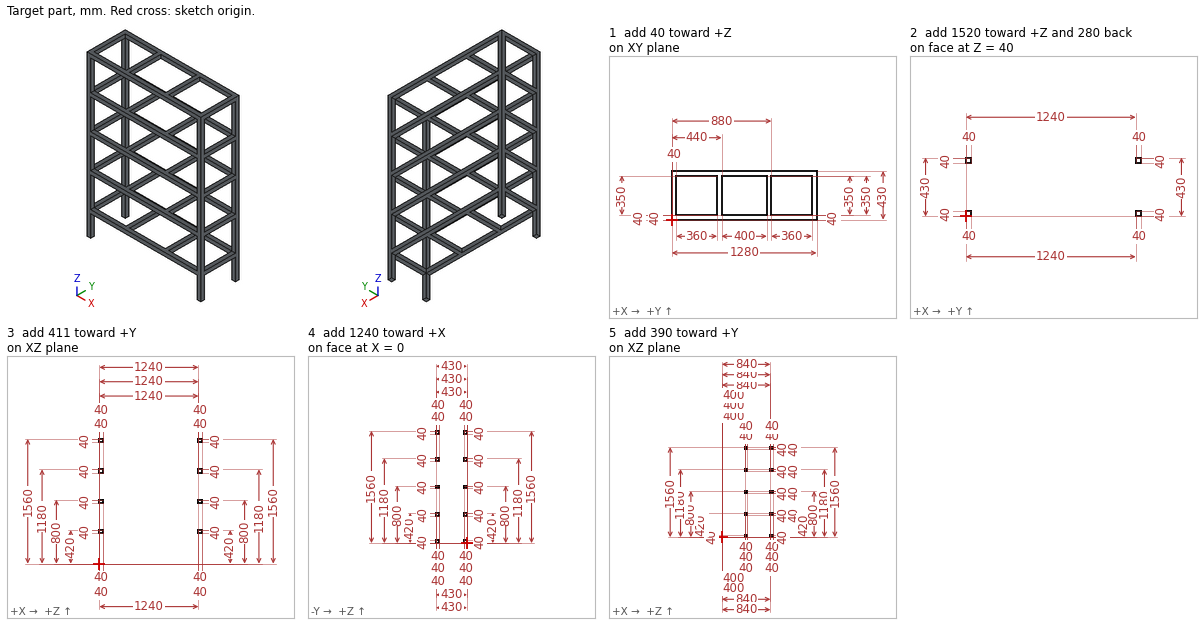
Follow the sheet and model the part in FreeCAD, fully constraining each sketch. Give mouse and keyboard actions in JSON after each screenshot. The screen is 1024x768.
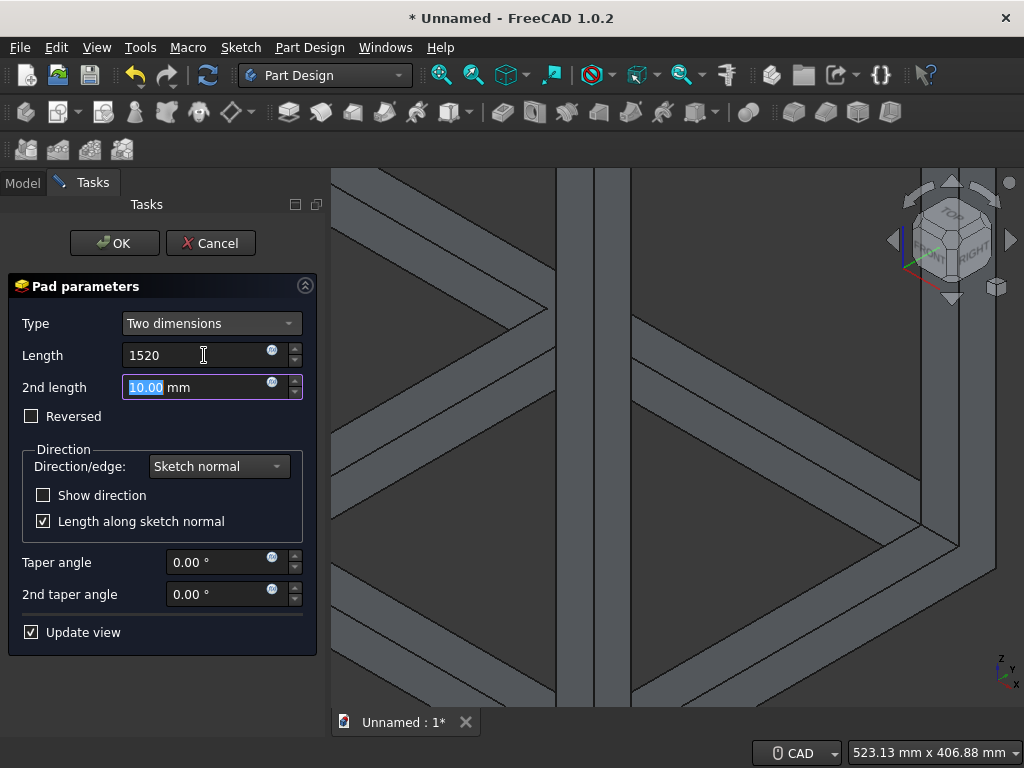
{"action": "type", "text": "280"}
{"action": "key", "text": "Tab"}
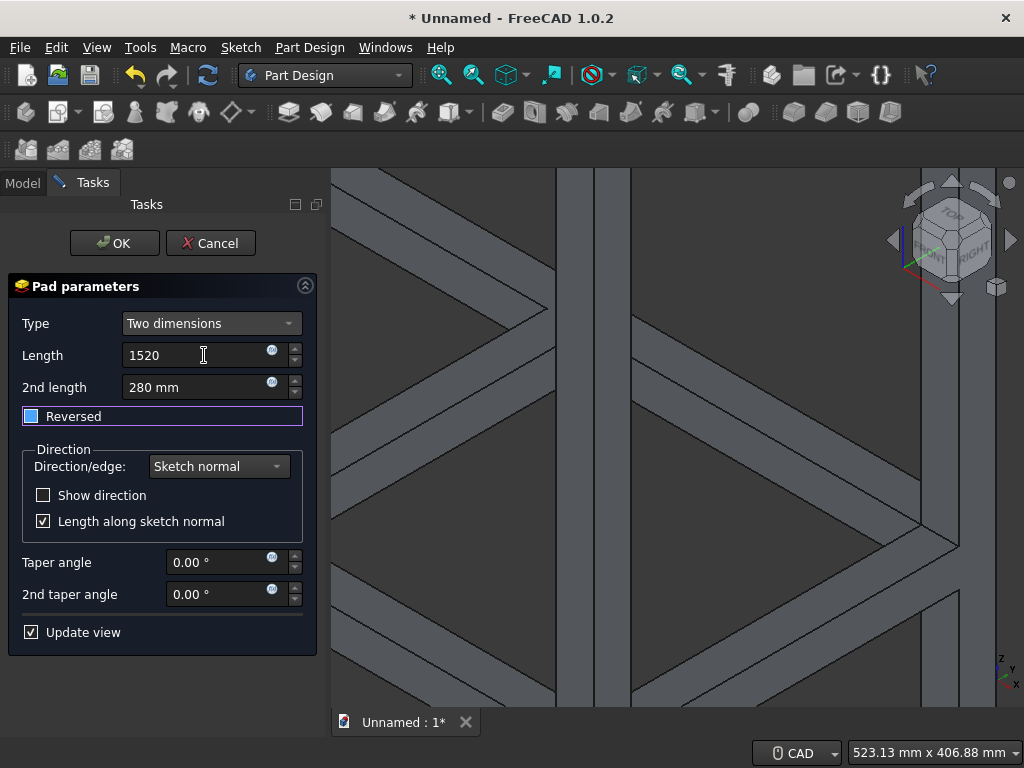
{"action": "left_click", "coordinate": [115, 243]}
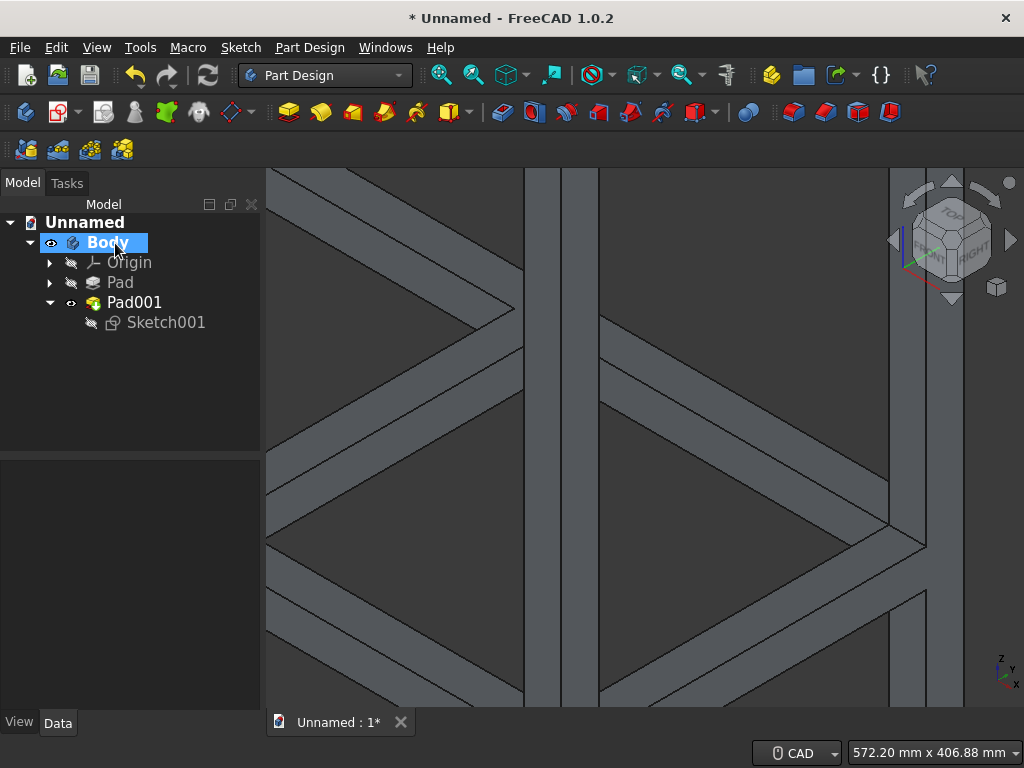
{"action": "left_click", "coordinate": [442, 76]}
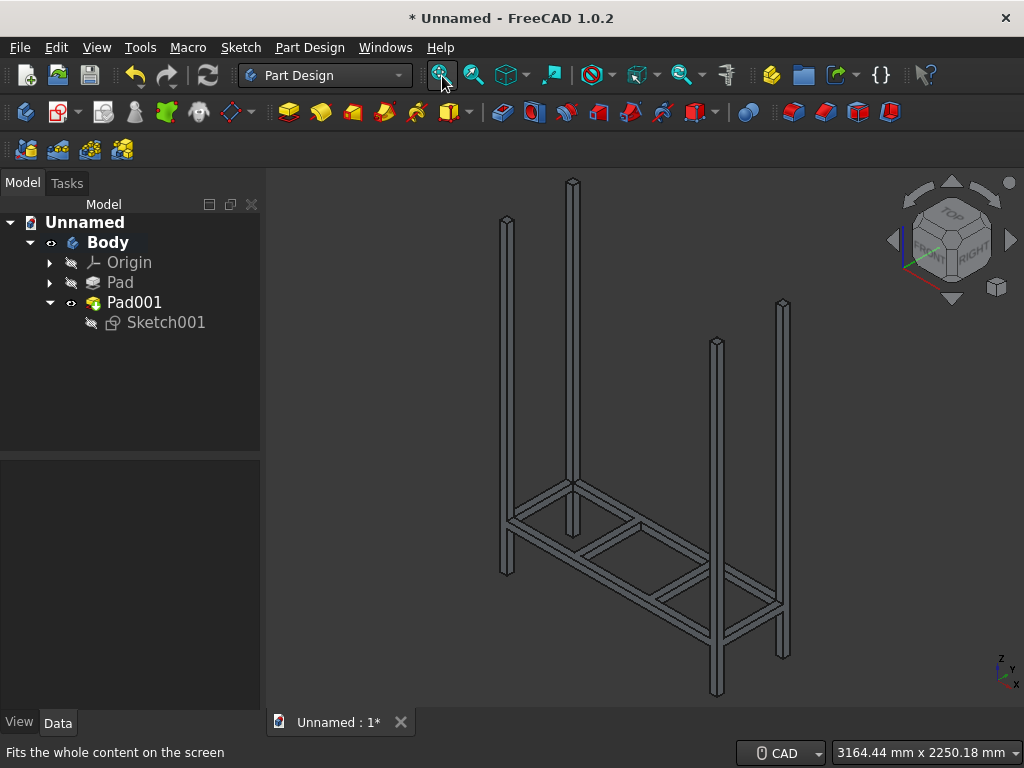
{"action": "left_click", "coordinate": [58, 112]}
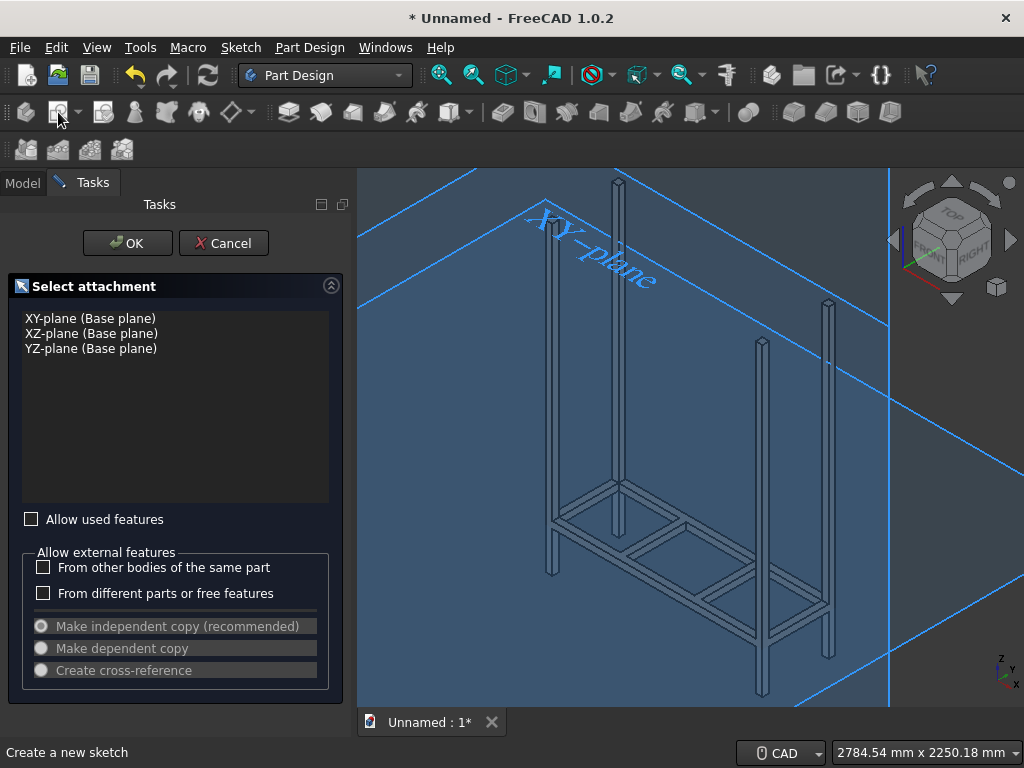
{"action": "left_click", "coordinate": [82, 334]}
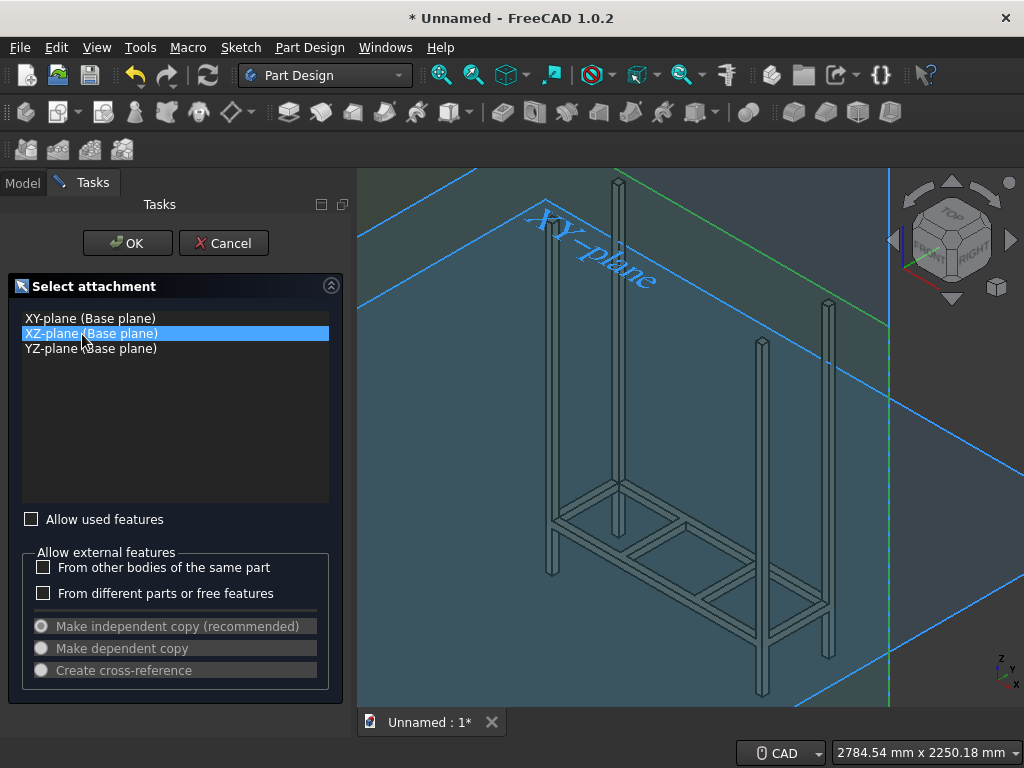
{"action": "left_click", "coordinate": [128, 243]}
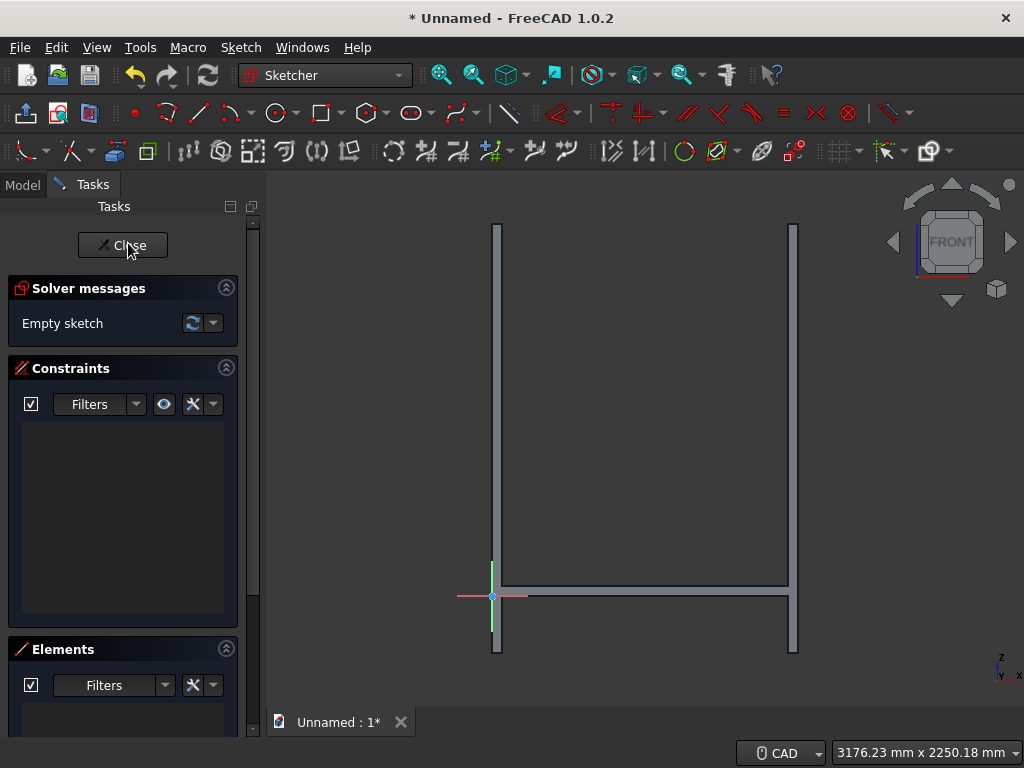
{"action": "left_click", "coordinate": [322, 114]}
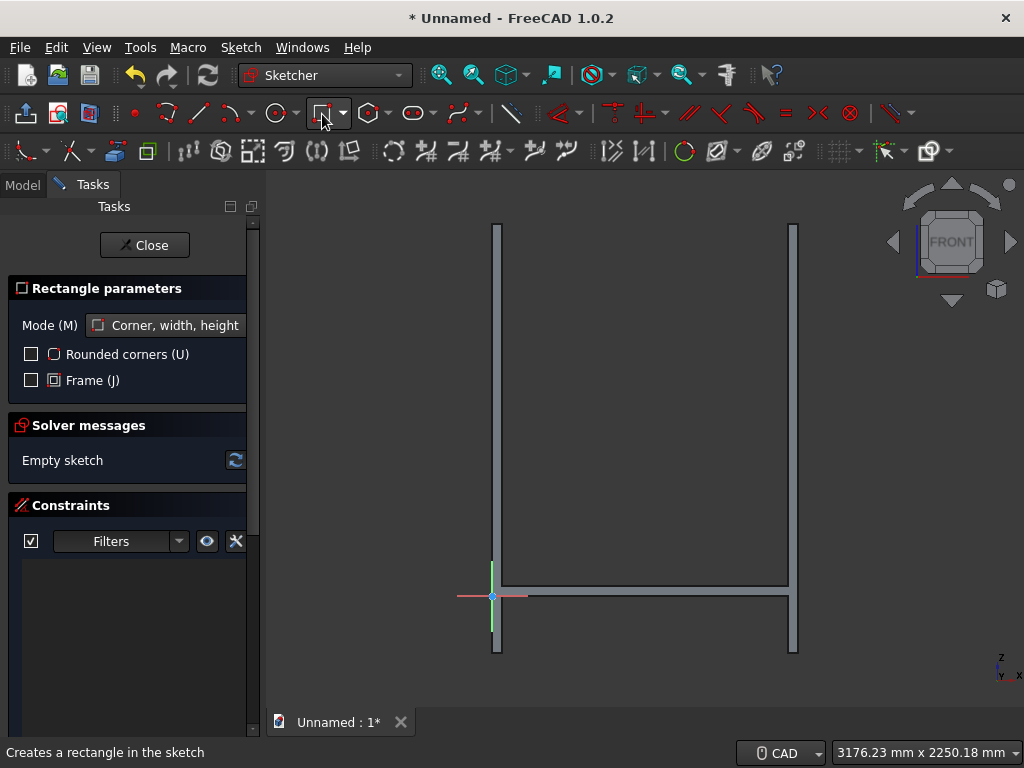
{"action": "scroll", "coordinate": [492, 496], "scroll_direction": "up", "scroll_amount": 3}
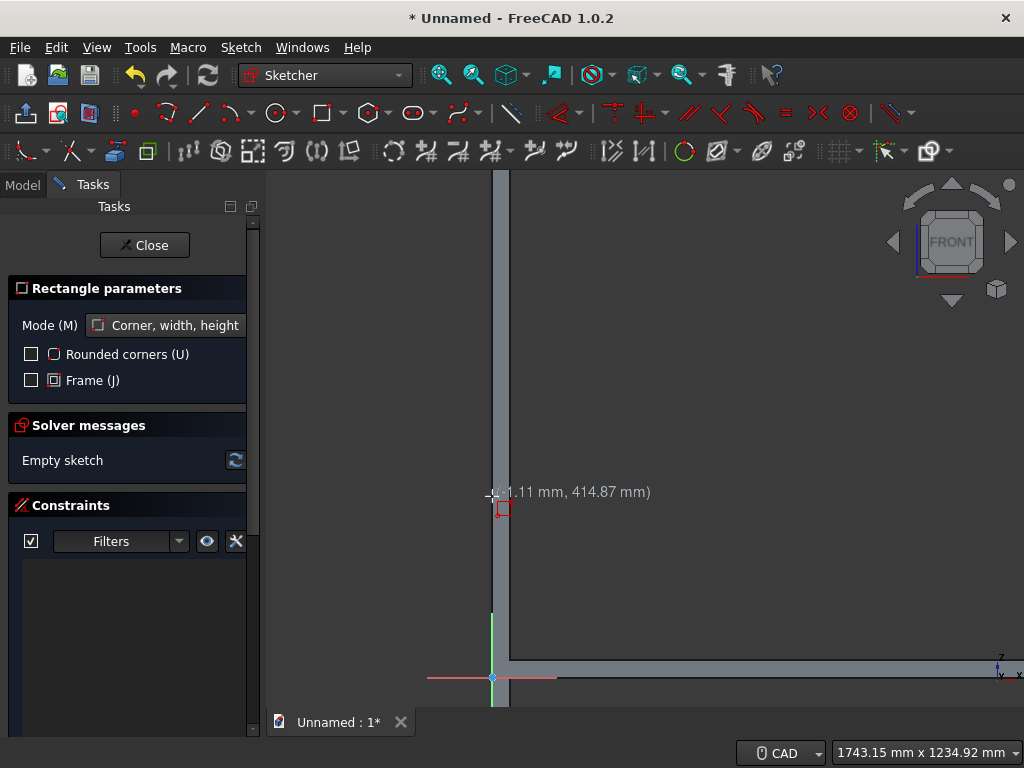
{"action": "left_click", "coordinate": [492, 495]}
{"action": "mouse_move", "coordinate": [510, 512]}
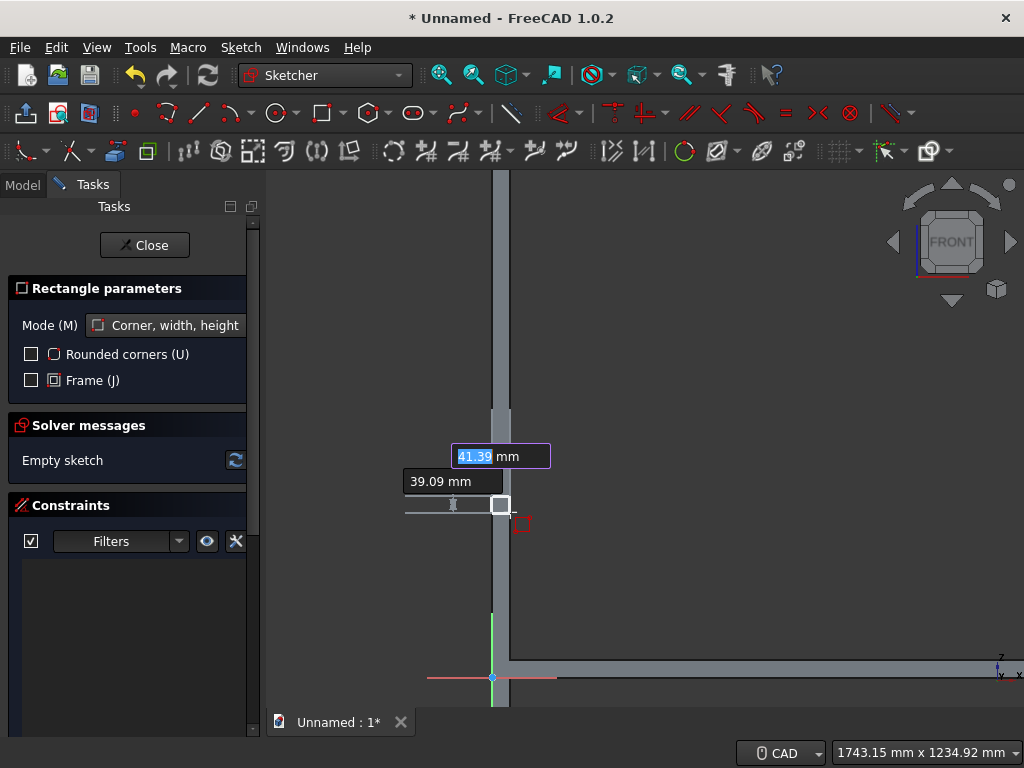
{"action": "type", "text": "40"}
{"action": "key", "text": "Tab"}
{"action": "type", "text": "40"}
{"action": "key", "text": "Return"}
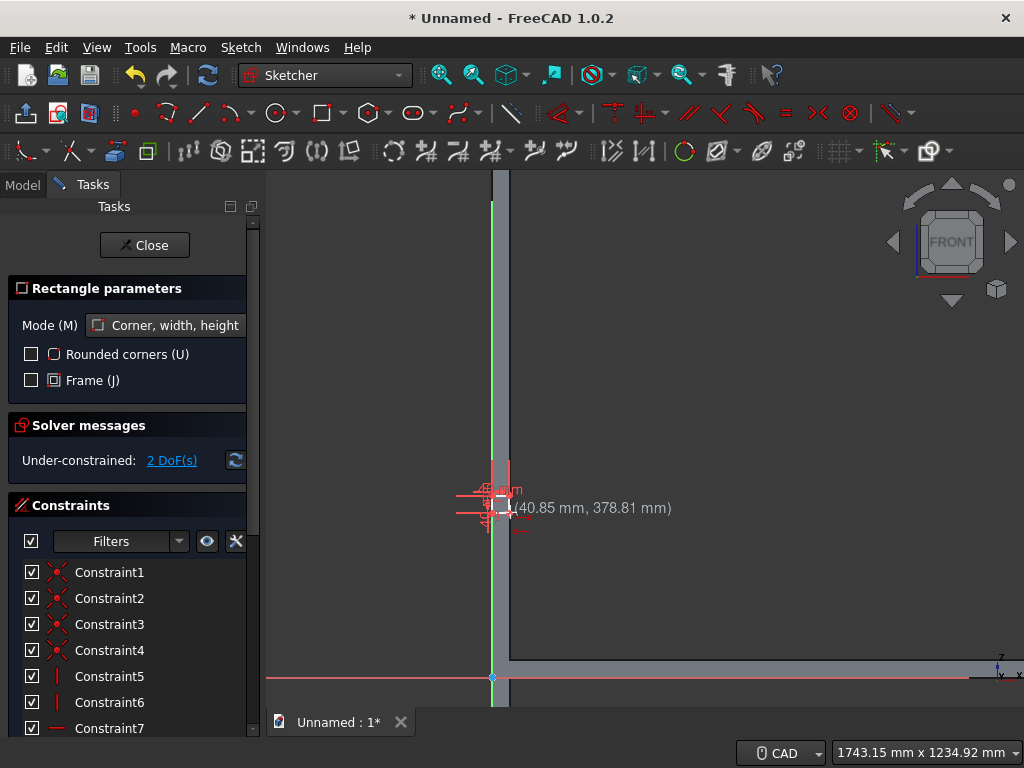
{"action": "scroll", "coordinate": [340, 560], "scroll_direction": "down", "scroll_amount": 3}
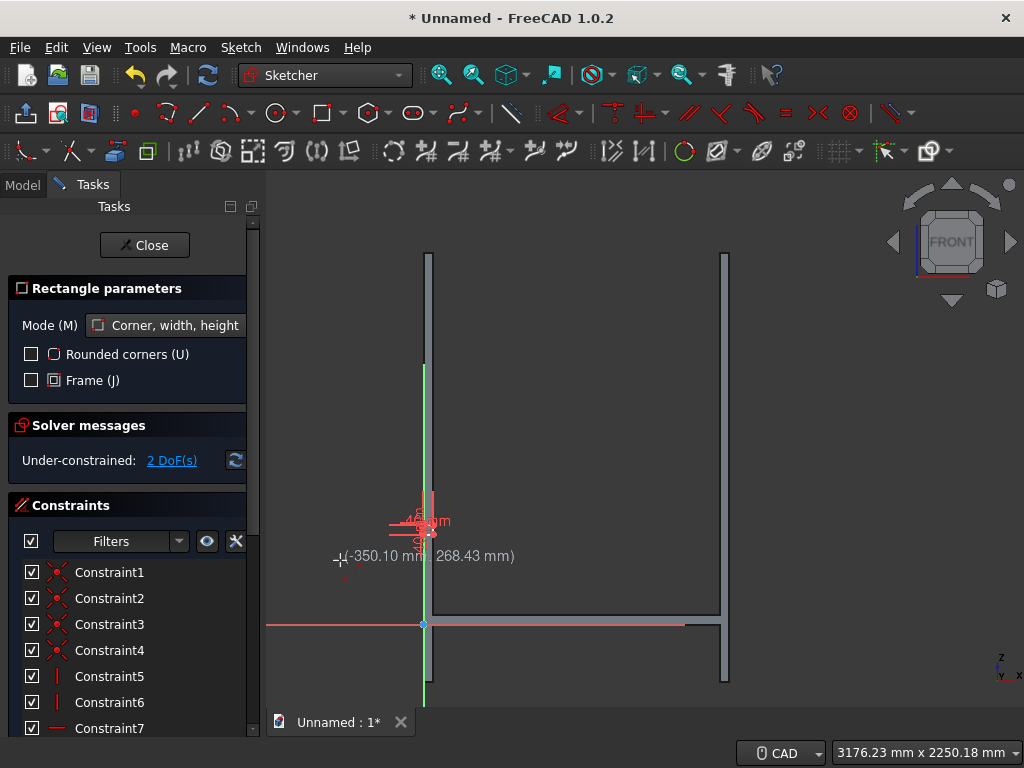
{"action": "scroll", "coordinate": [720, 525], "scroll_direction": "up", "scroll_amount": 3}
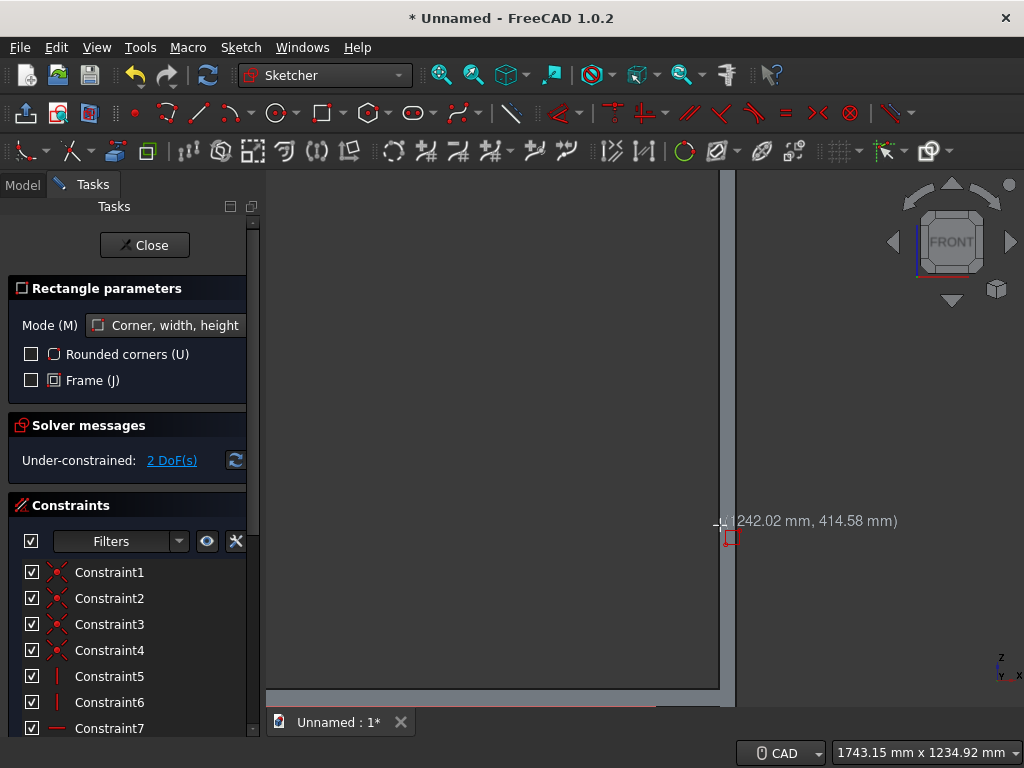
{"action": "left_click", "coordinate": [719, 524]}
{"action": "mouse_move", "coordinate": [736, 541]}